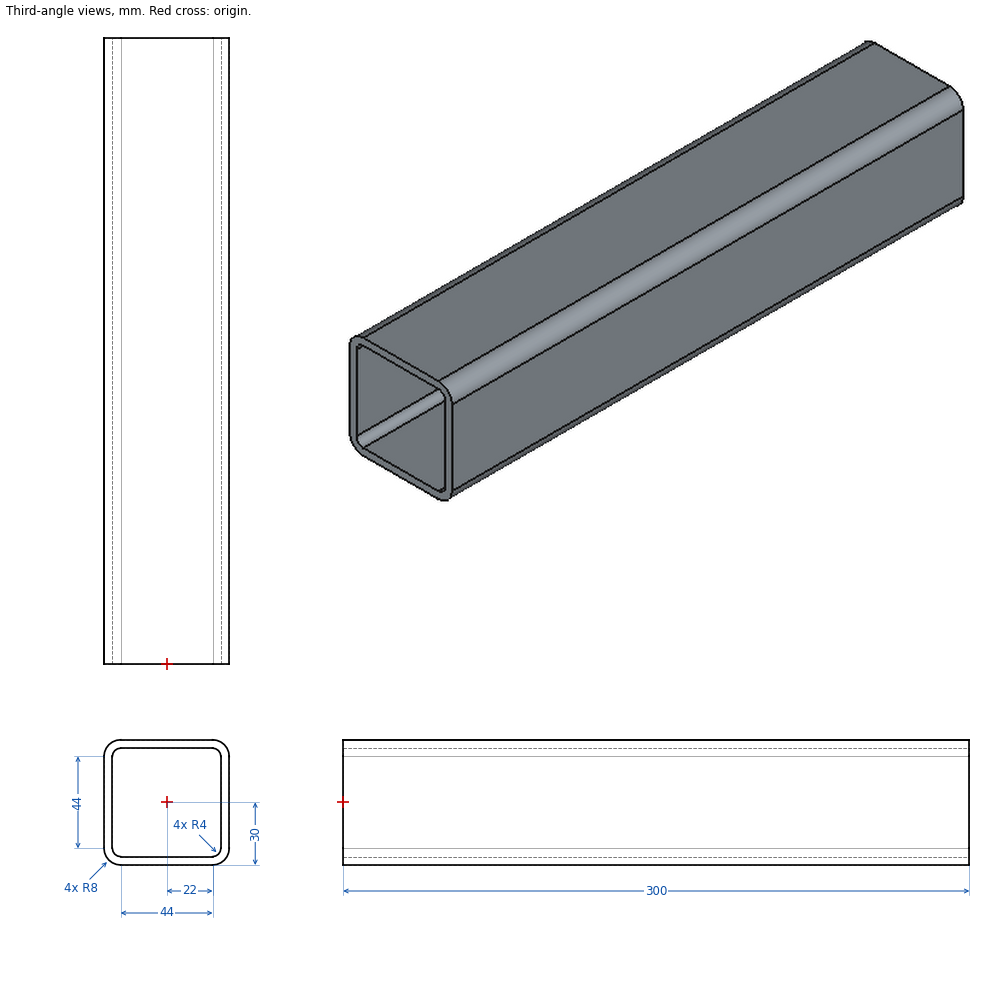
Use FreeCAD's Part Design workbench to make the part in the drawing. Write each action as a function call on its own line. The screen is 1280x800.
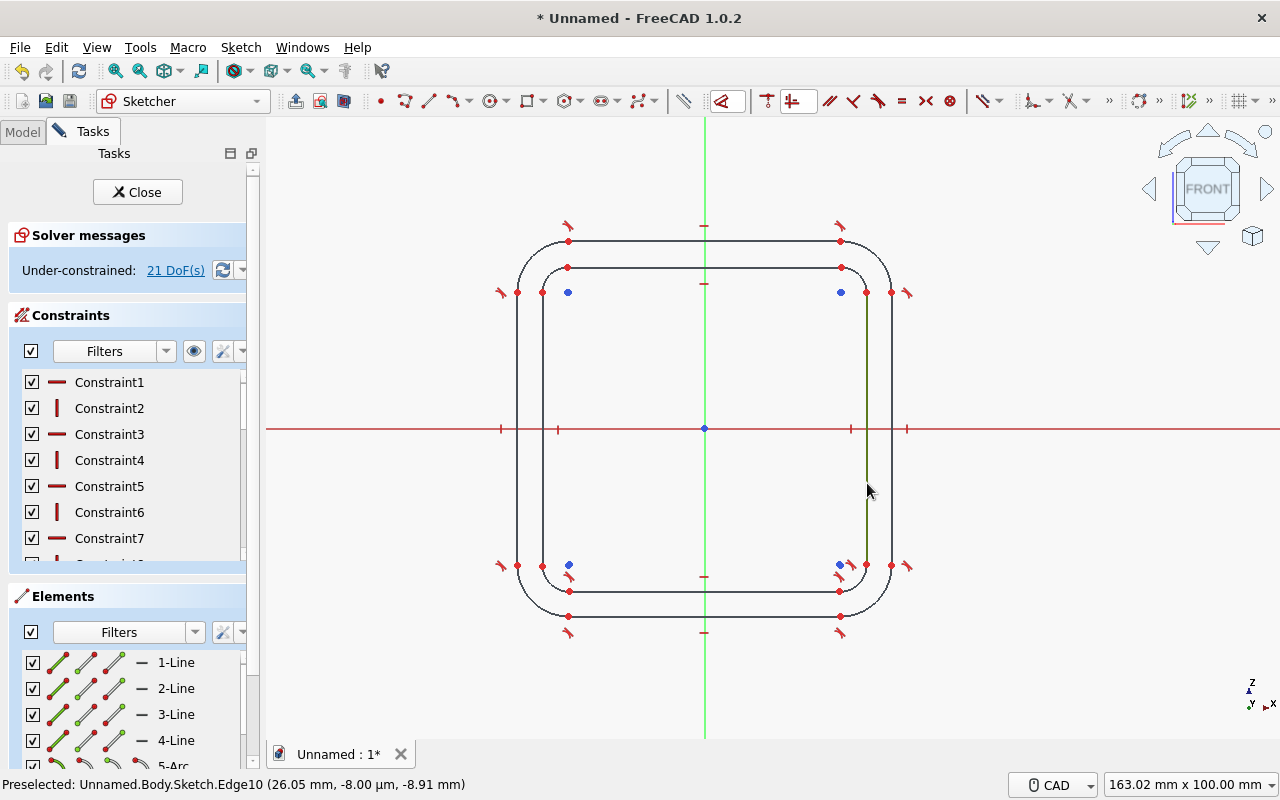
click(864, 281)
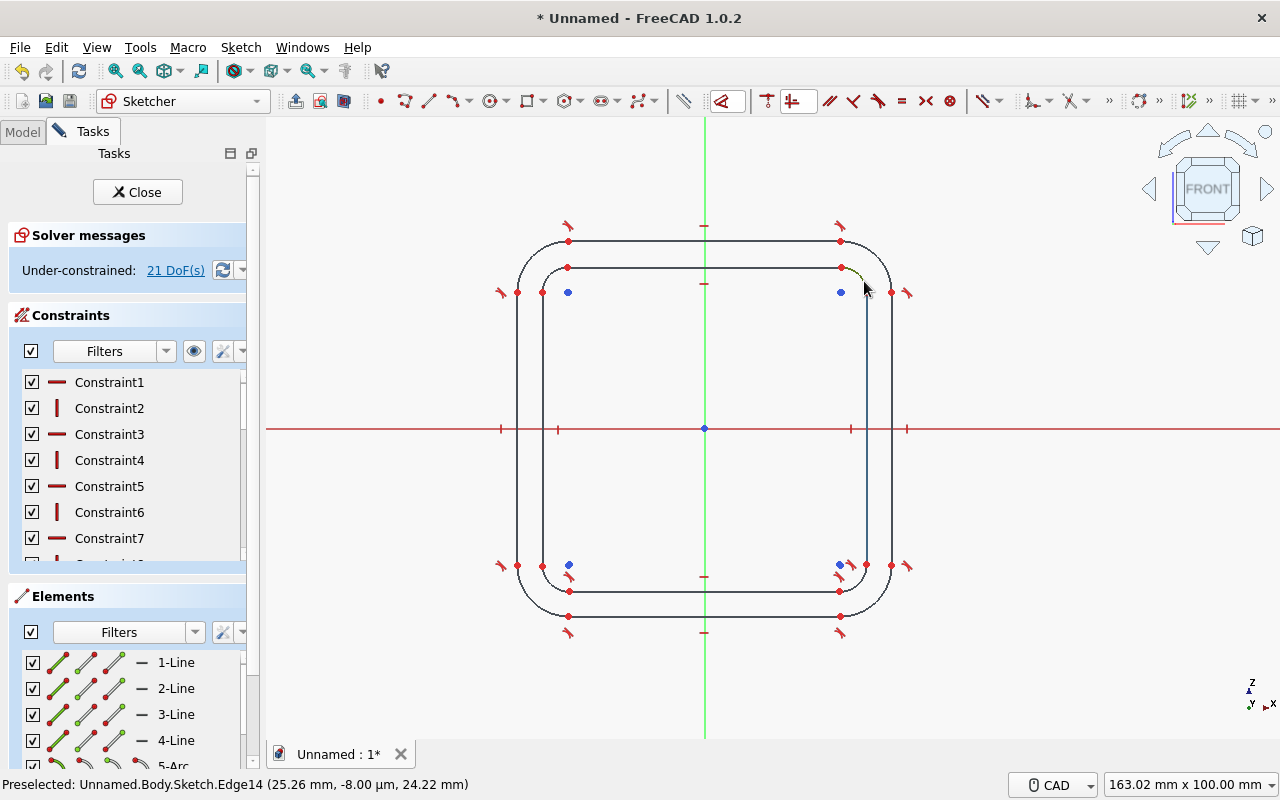
click(878, 102)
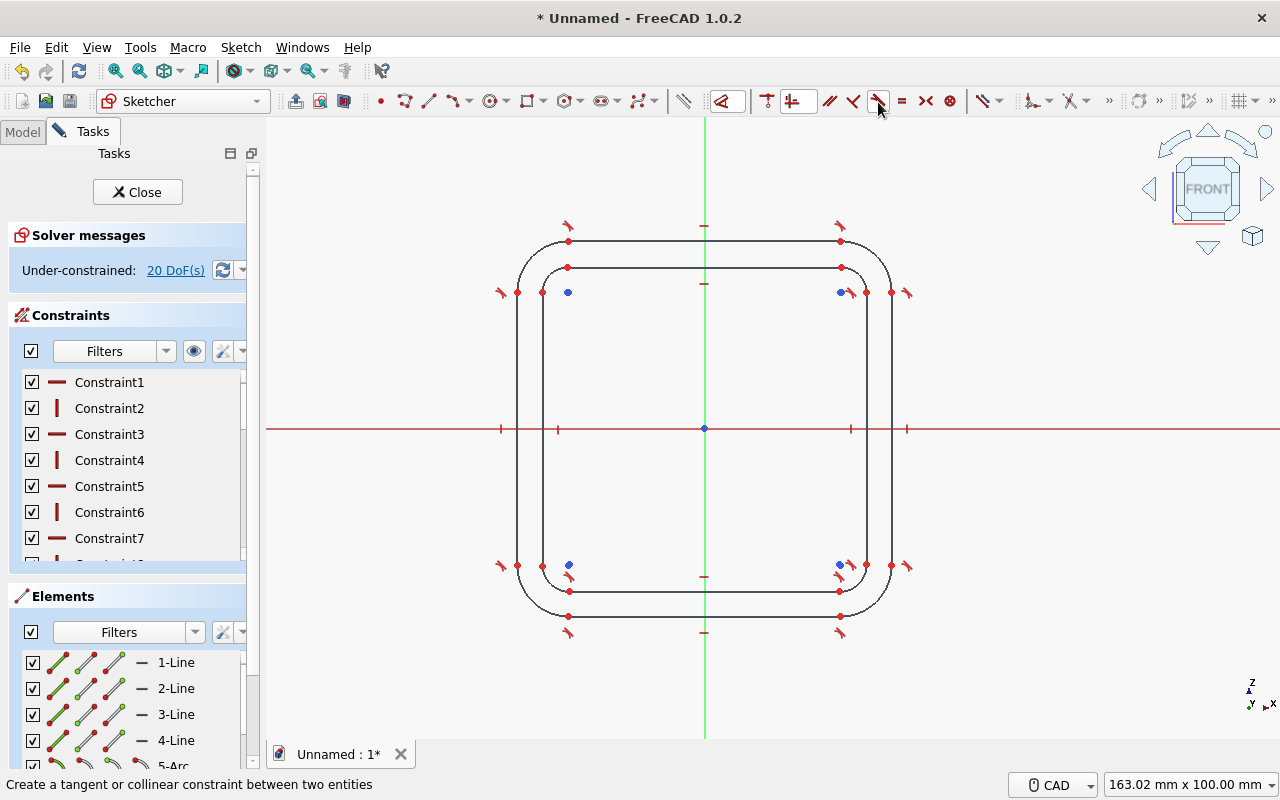
click(759, 268)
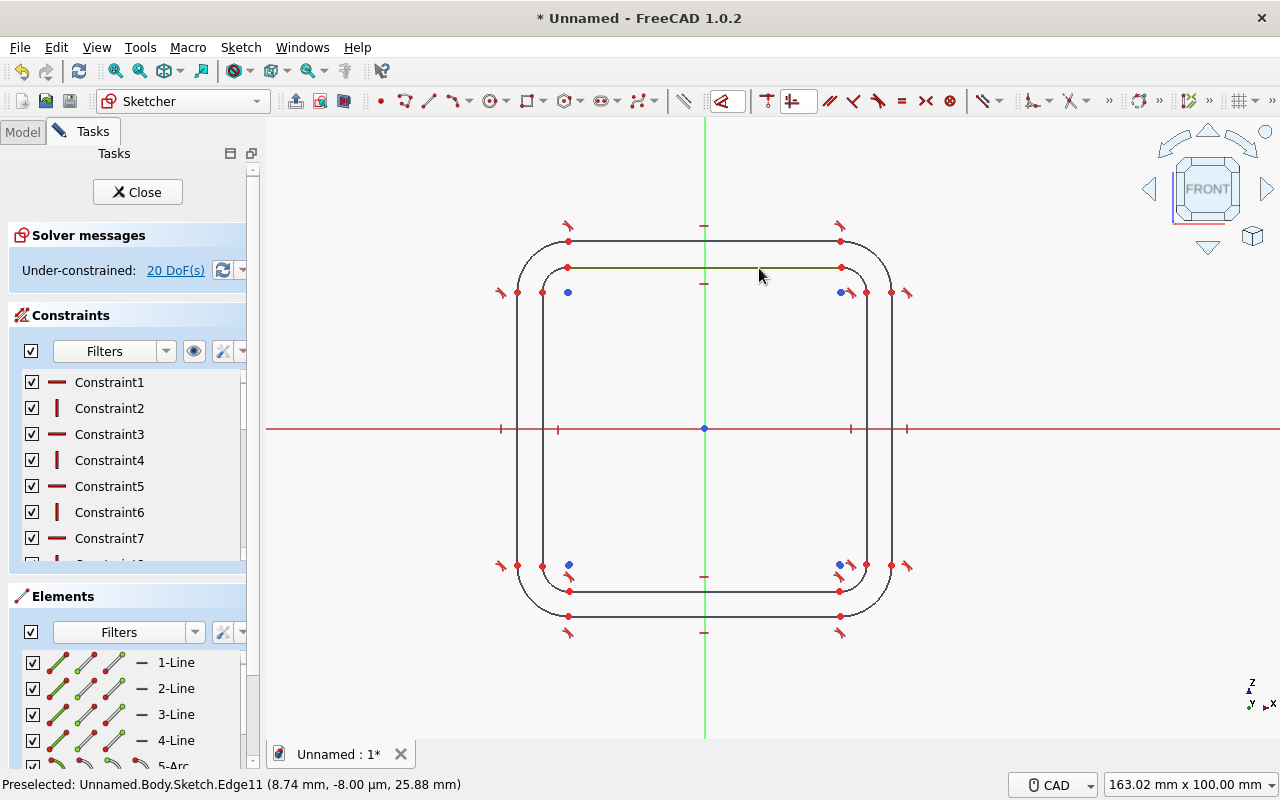
click(864, 281)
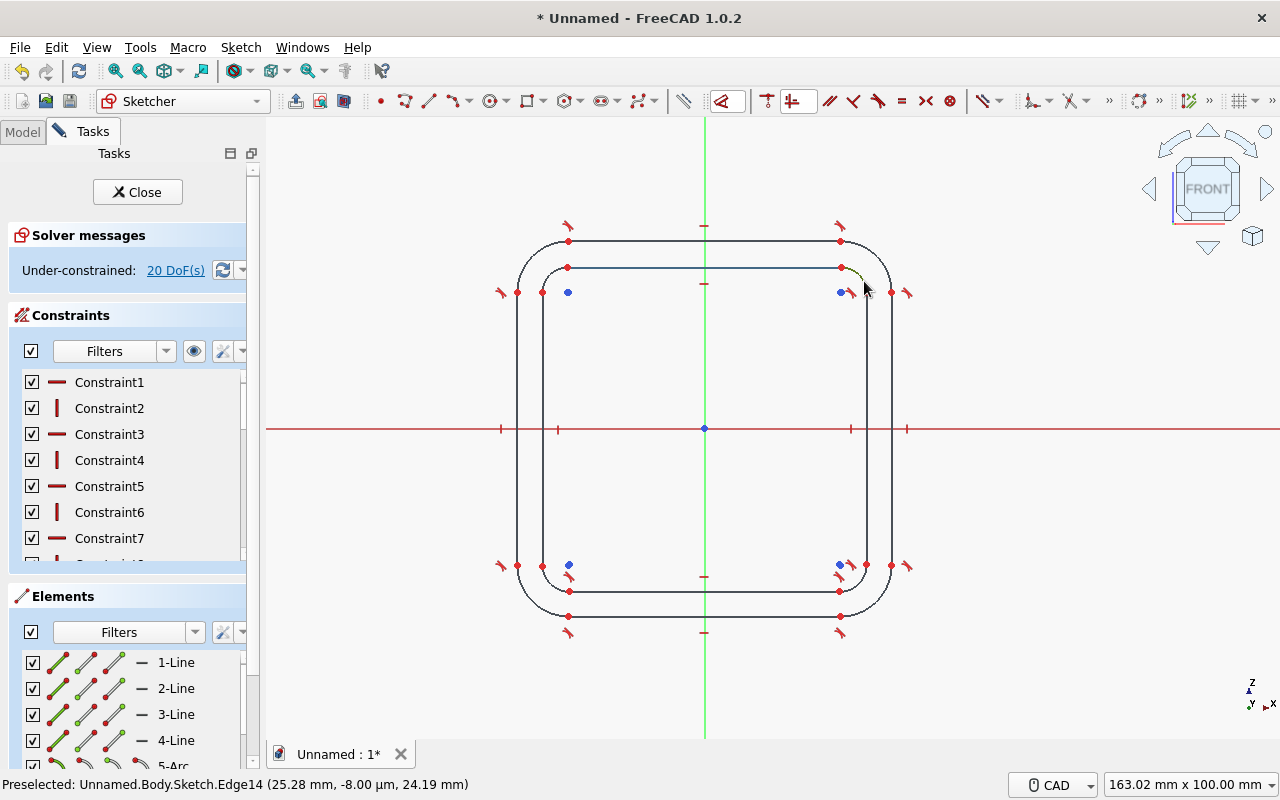
click(878, 102)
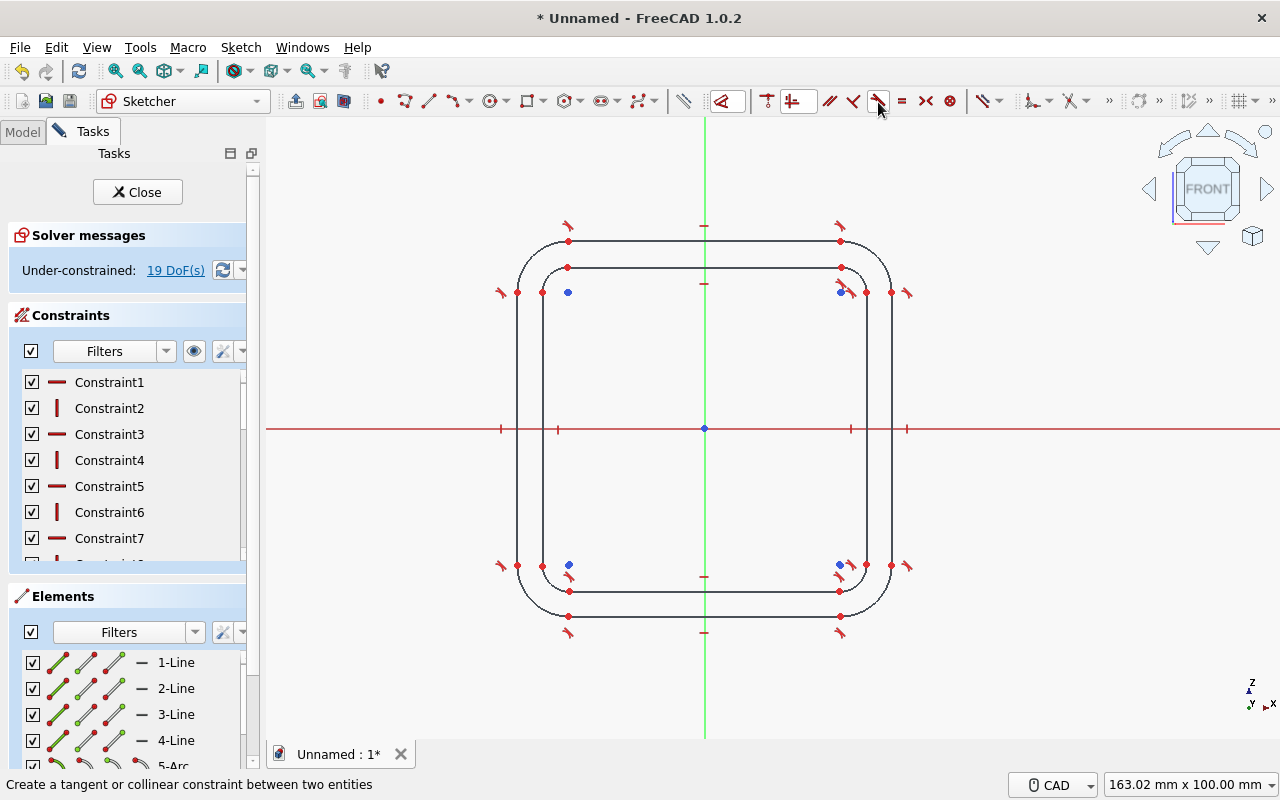
click(759, 268)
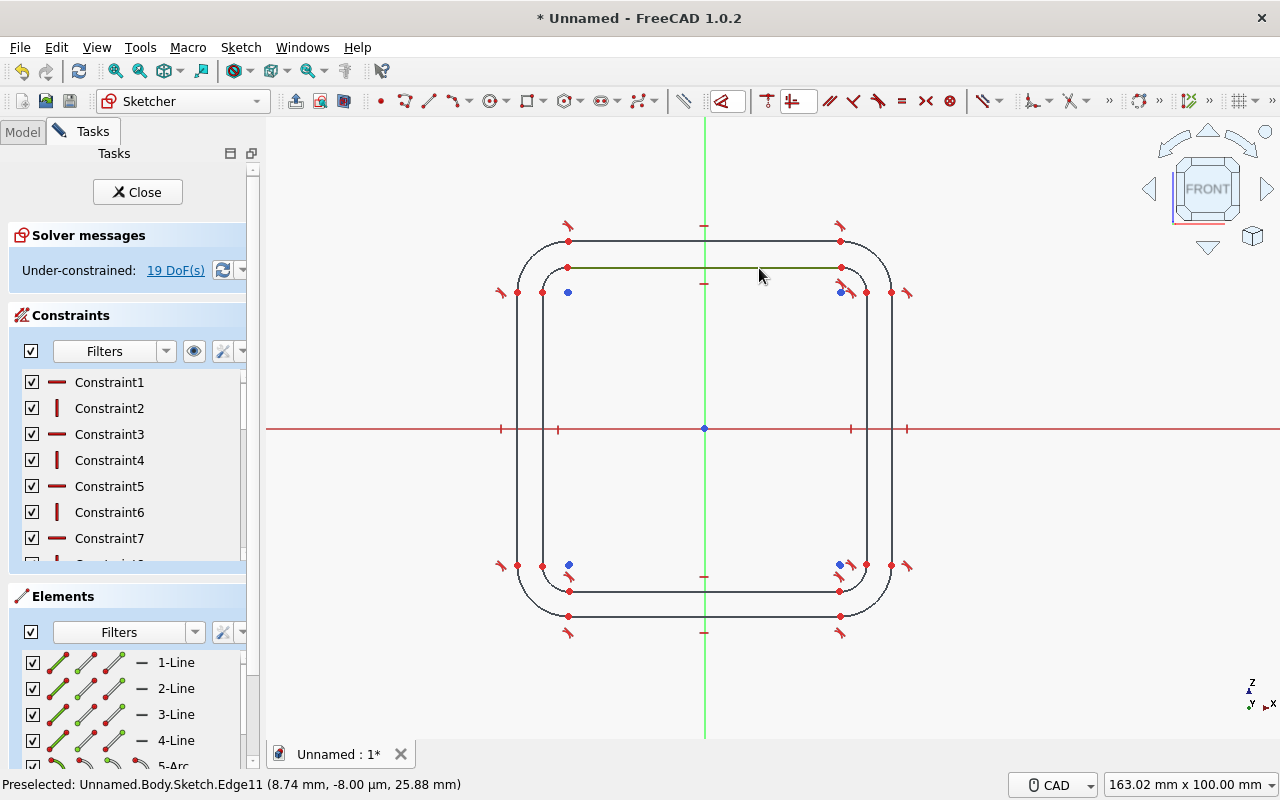
click(556, 270)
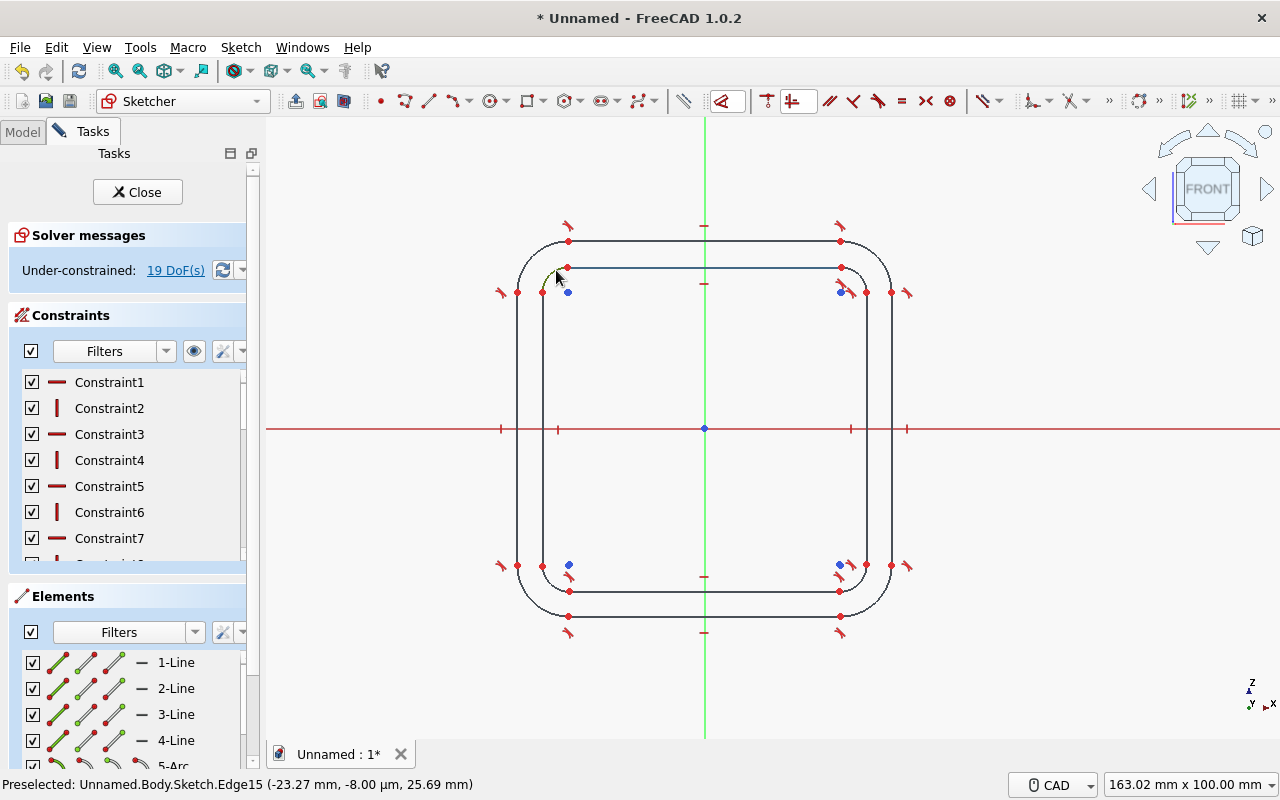
click(878, 102)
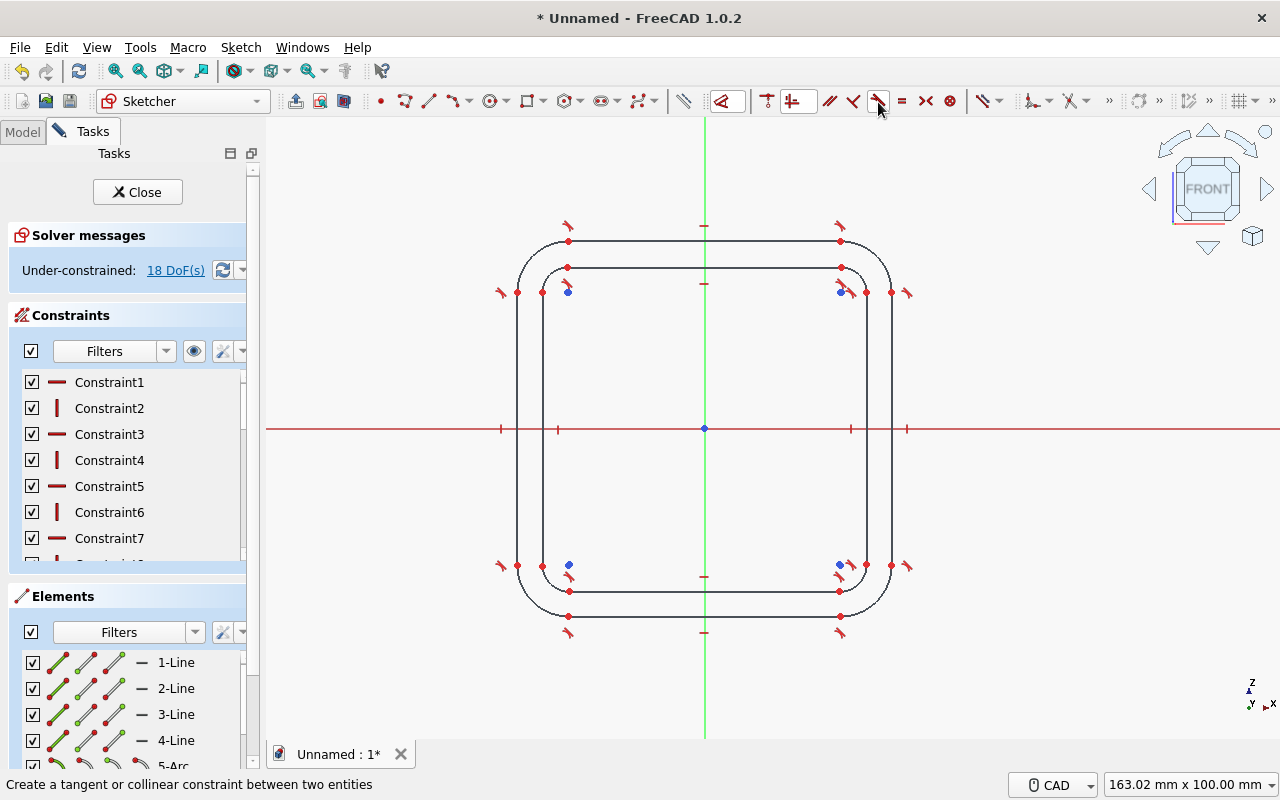
click(543, 375)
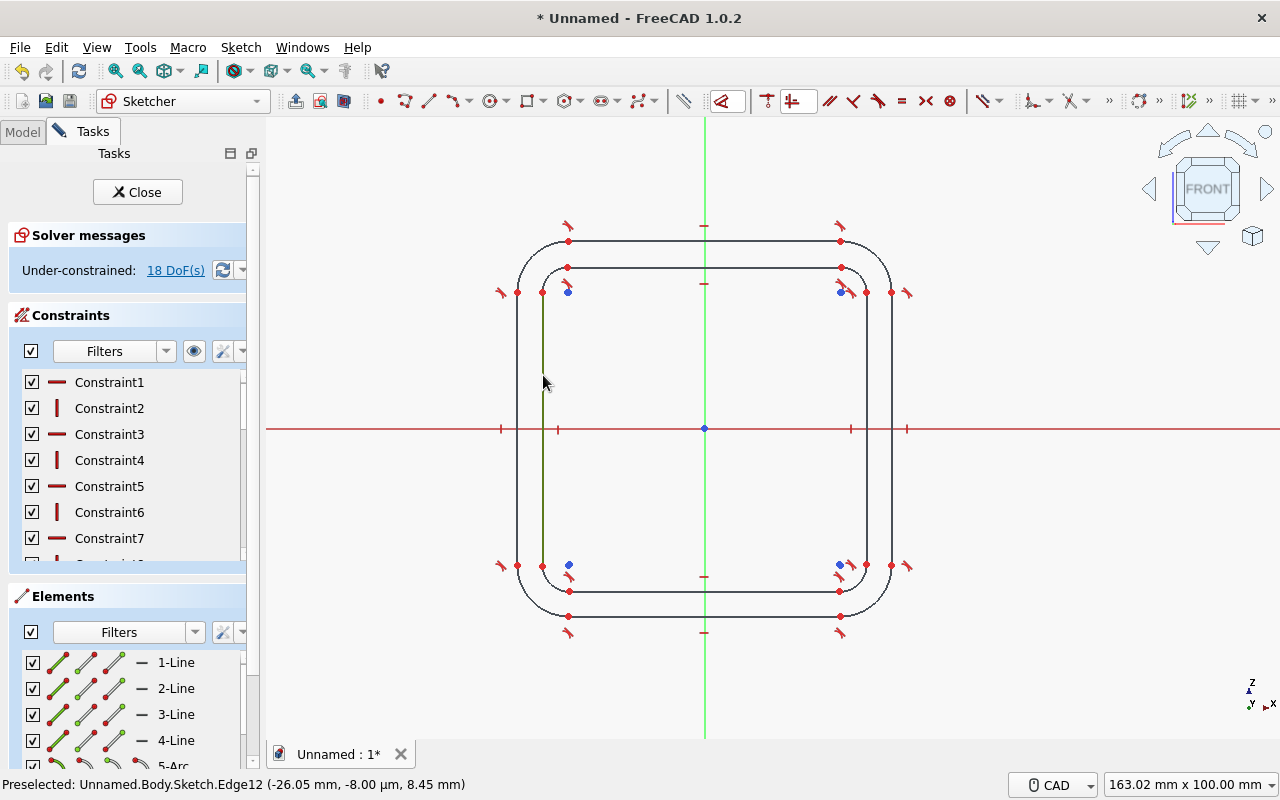
click(556, 270)